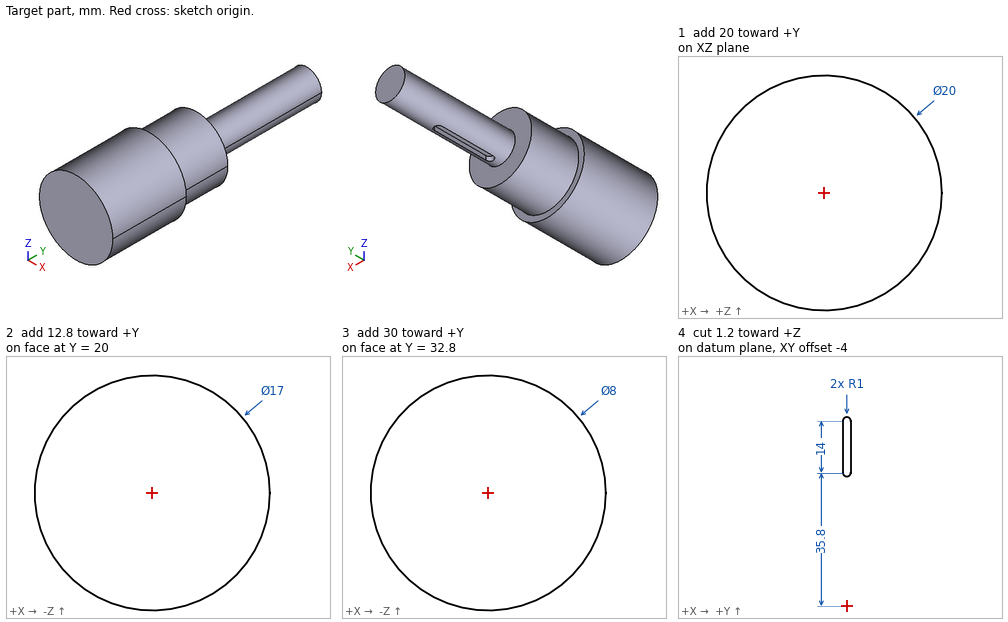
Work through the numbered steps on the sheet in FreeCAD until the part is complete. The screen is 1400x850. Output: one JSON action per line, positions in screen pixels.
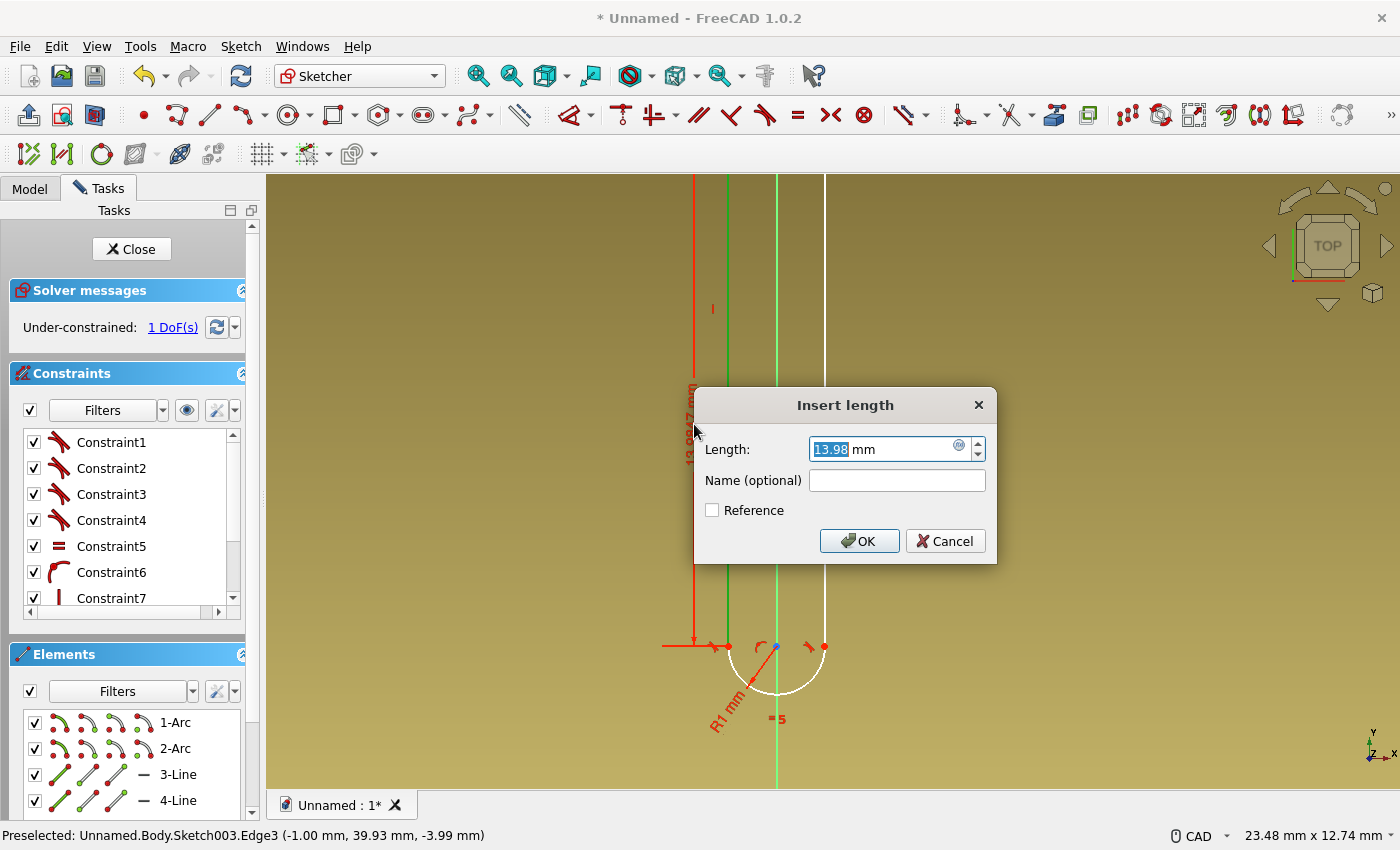
{"action": "type", "text": "14"}
{"action": "key", "text": "Return"}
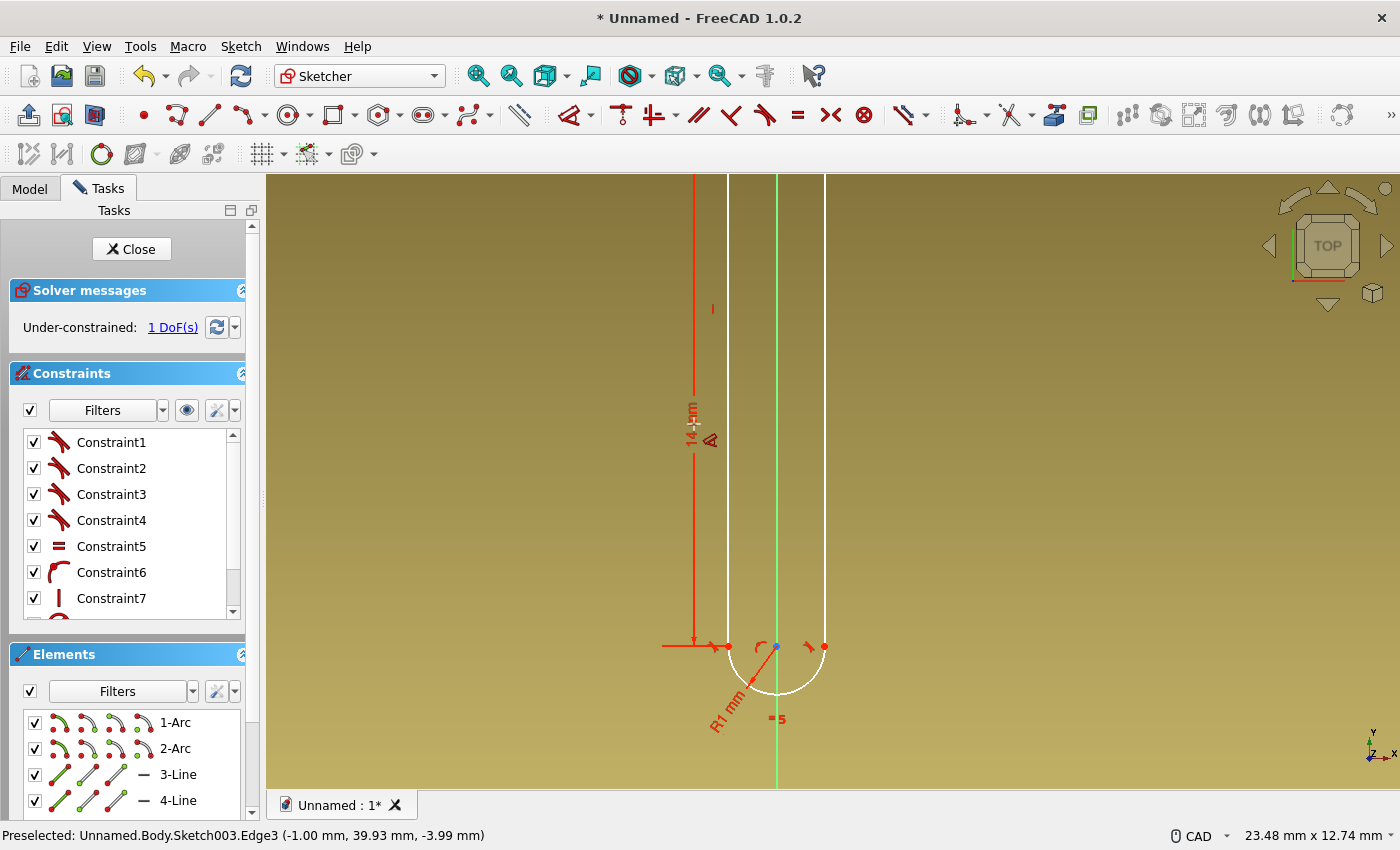
{"action": "left_click", "coordinate": [728, 646]}
{"action": "left_click", "coordinate": [694, 677]}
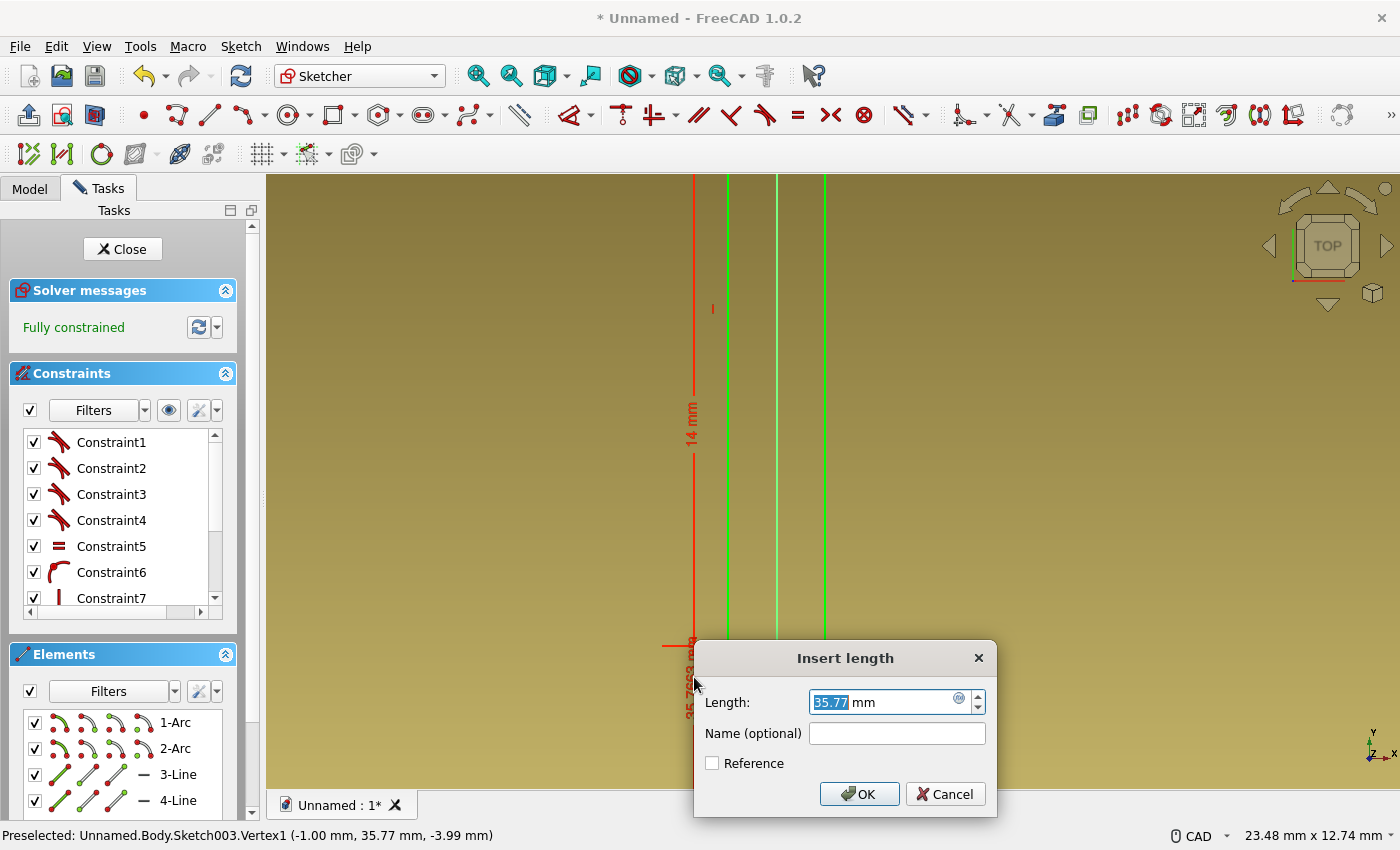
{"action": "type", "text": "35.8"}
{"action": "key", "text": "Return"}
{"action": "key", "text": "Escape"}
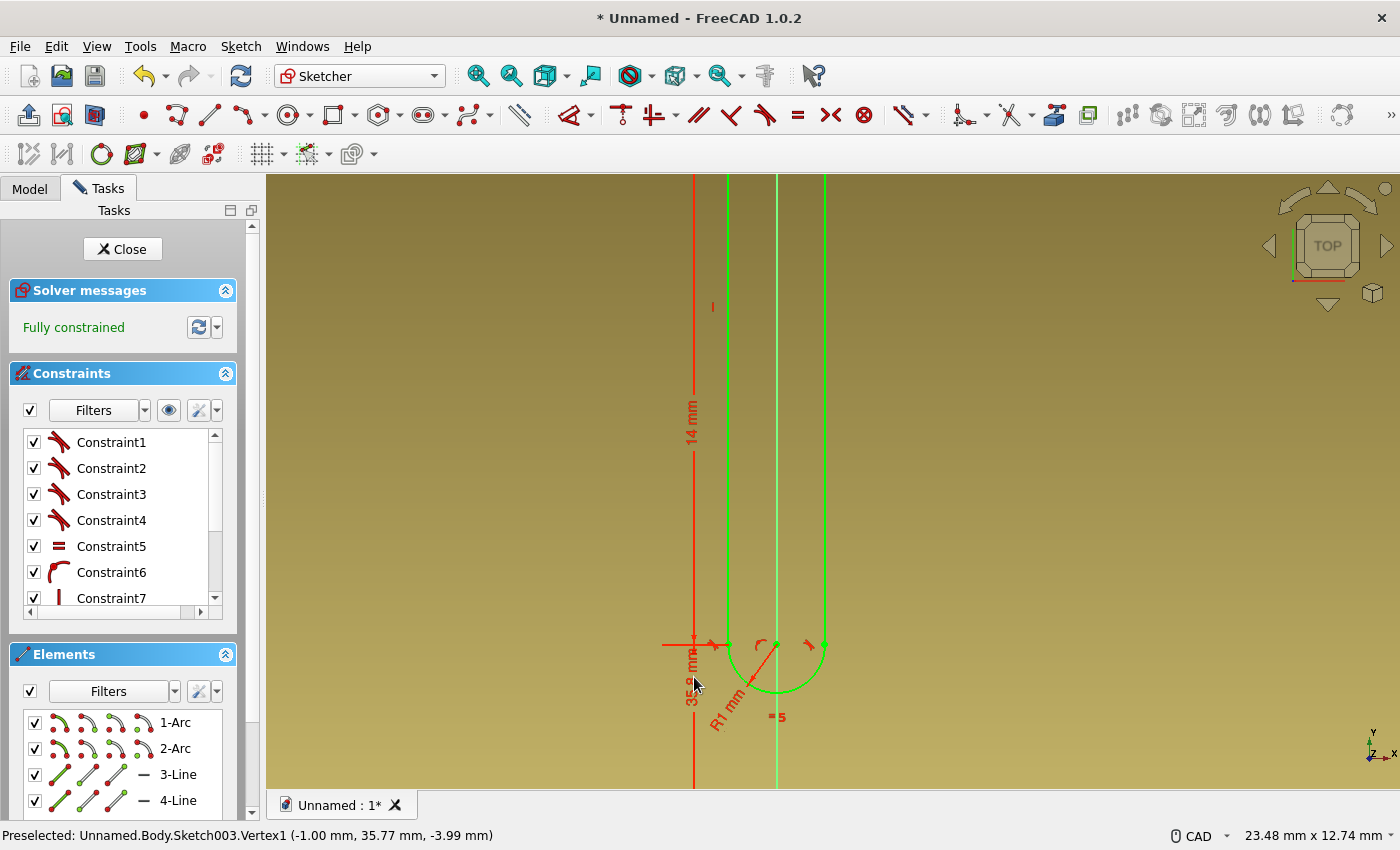
{"action": "left_click", "coordinate": [123, 249]}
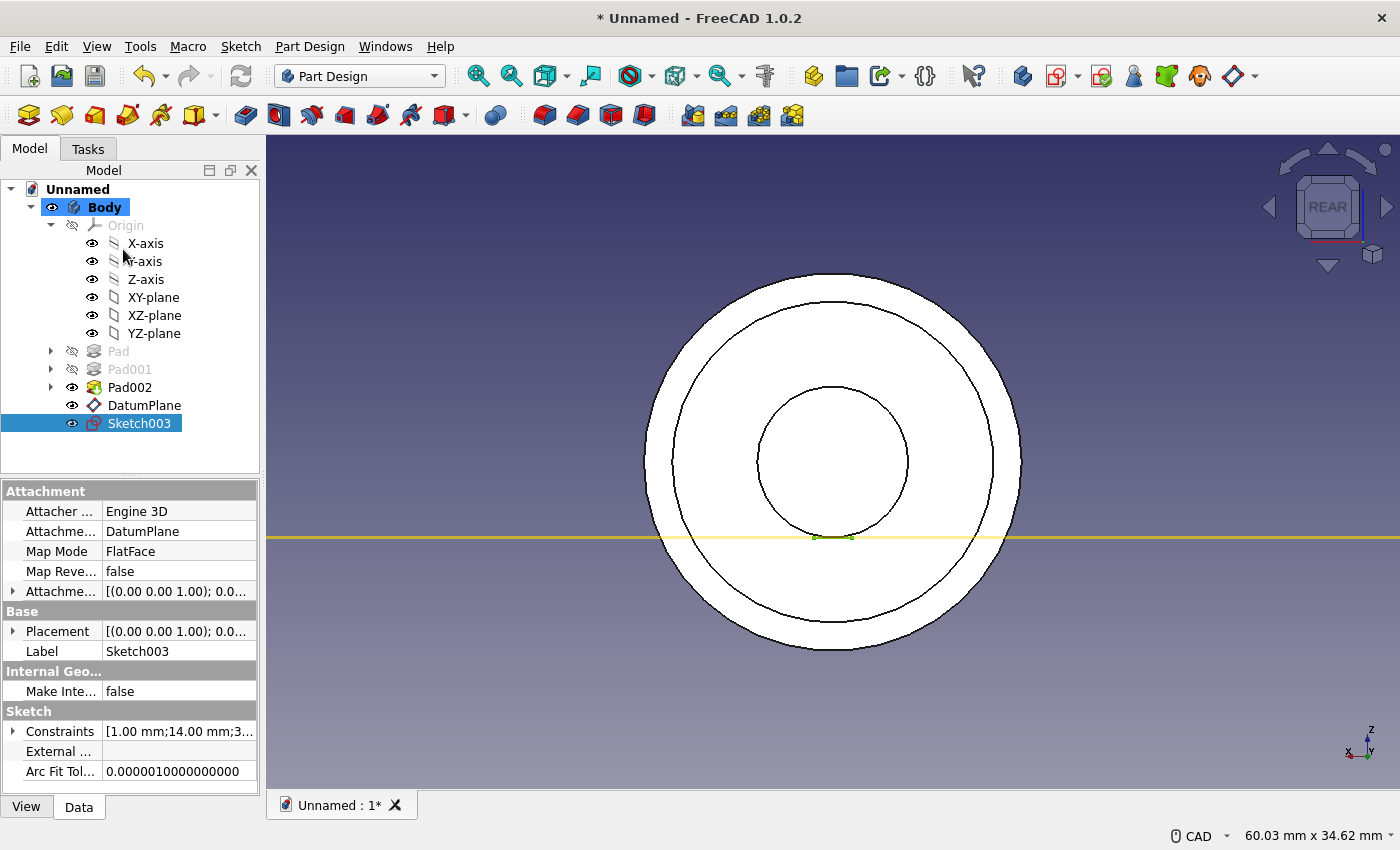
{"action": "left_click", "coordinate": [246, 116]}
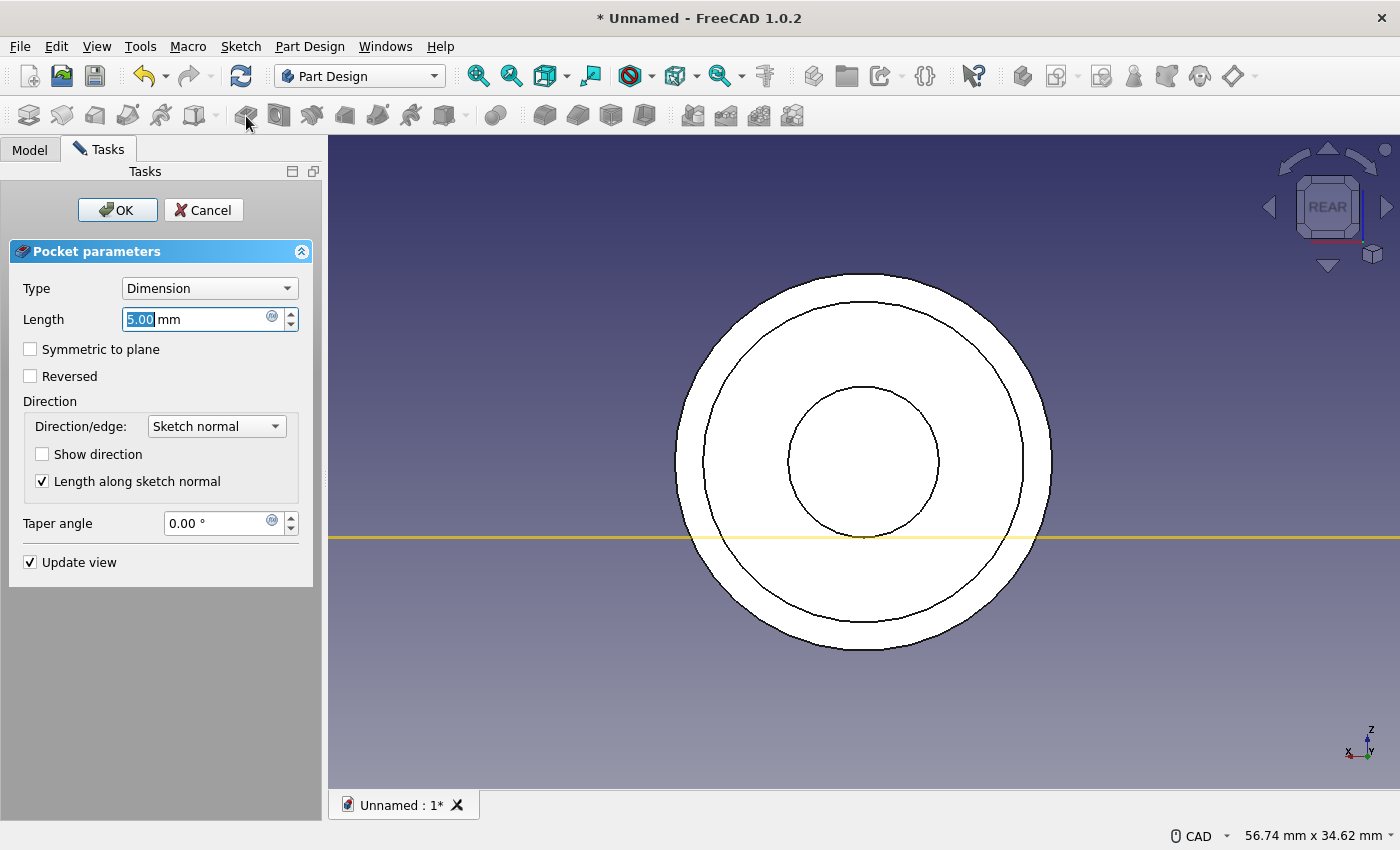
{"action": "type", "text": "1.2"}
{"action": "key", "text": "Tab"}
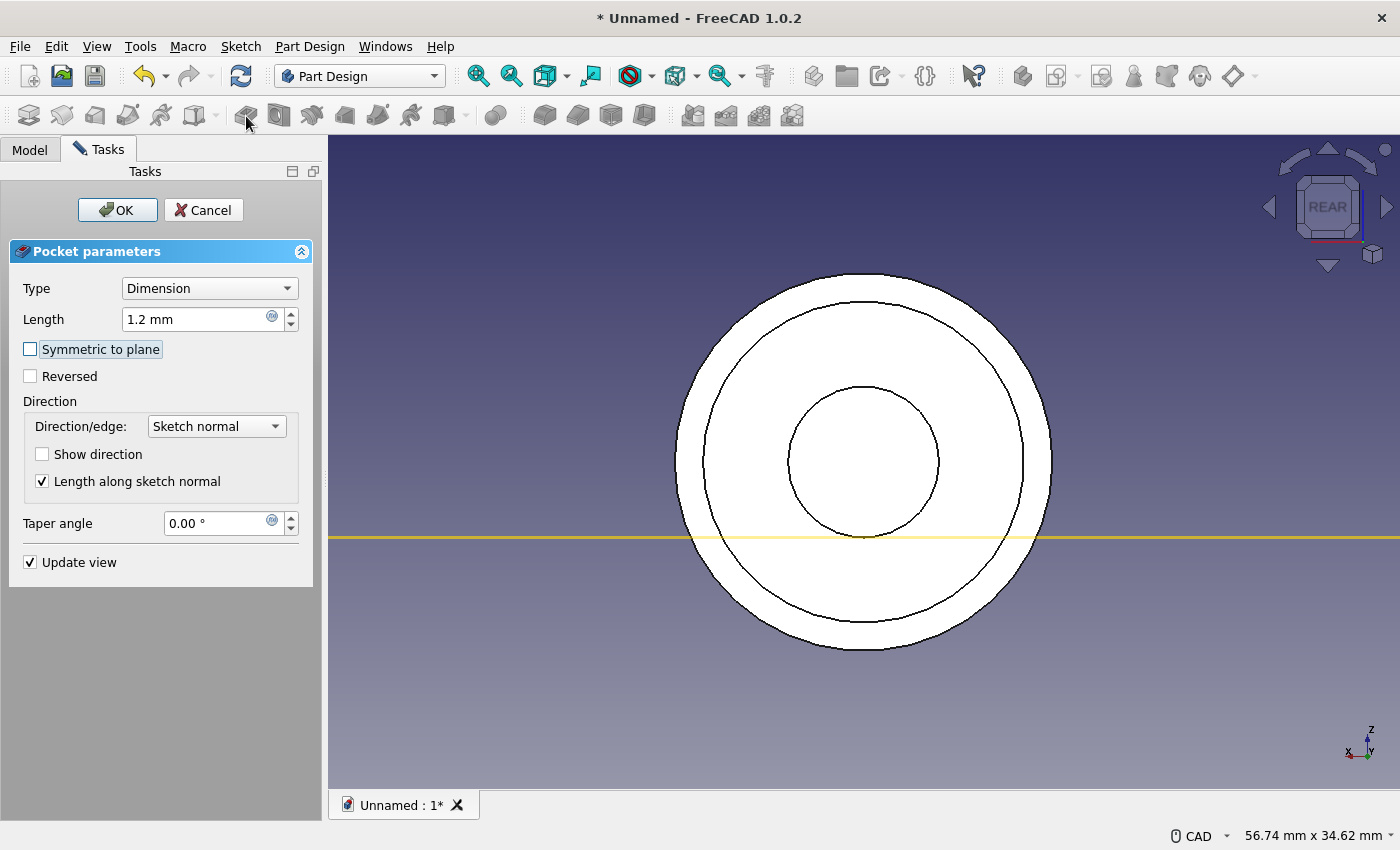
{"action": "left_click", "coordinate": [31, 376]}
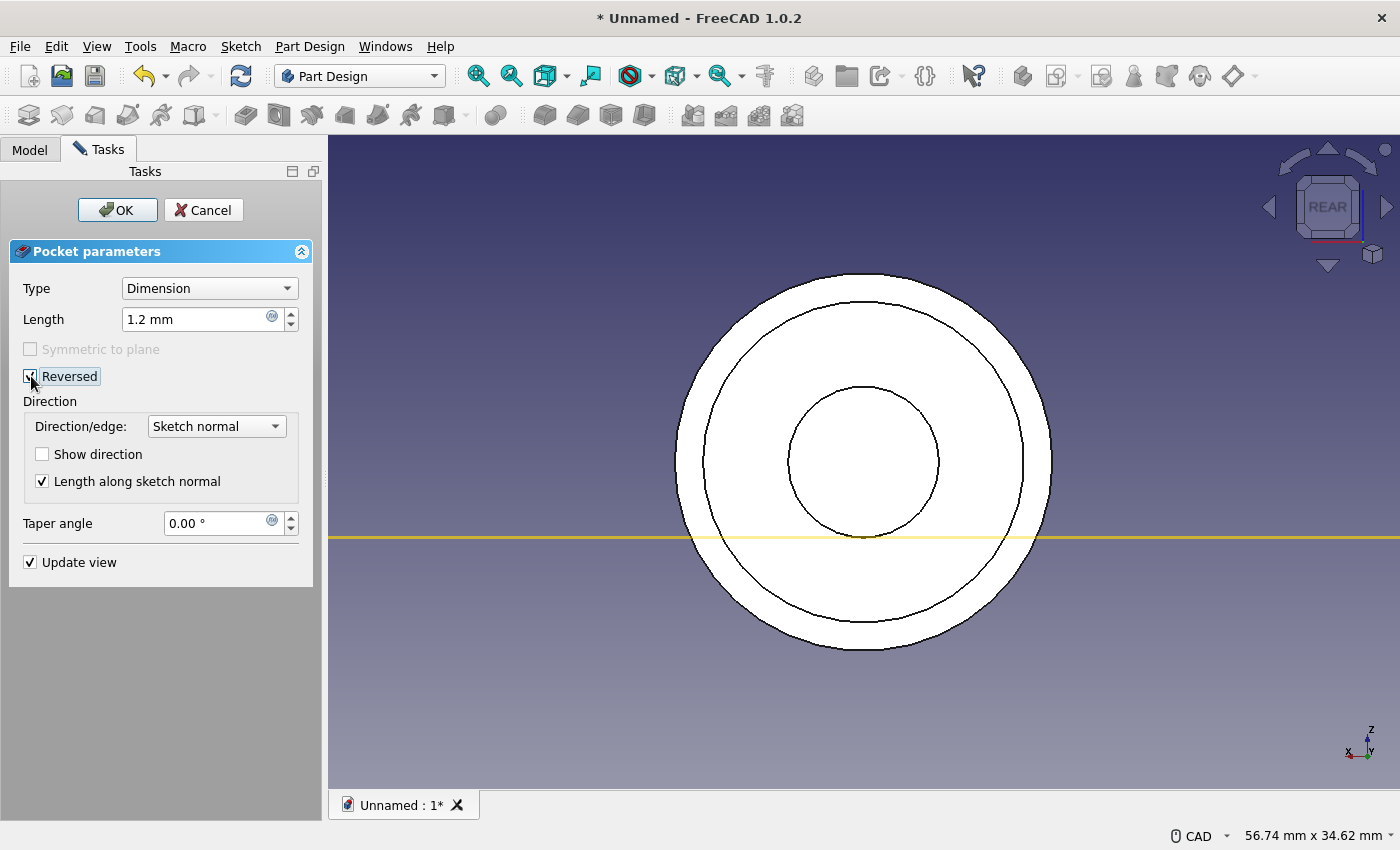
{"action": "left_click", "coordinate": [118, 210]}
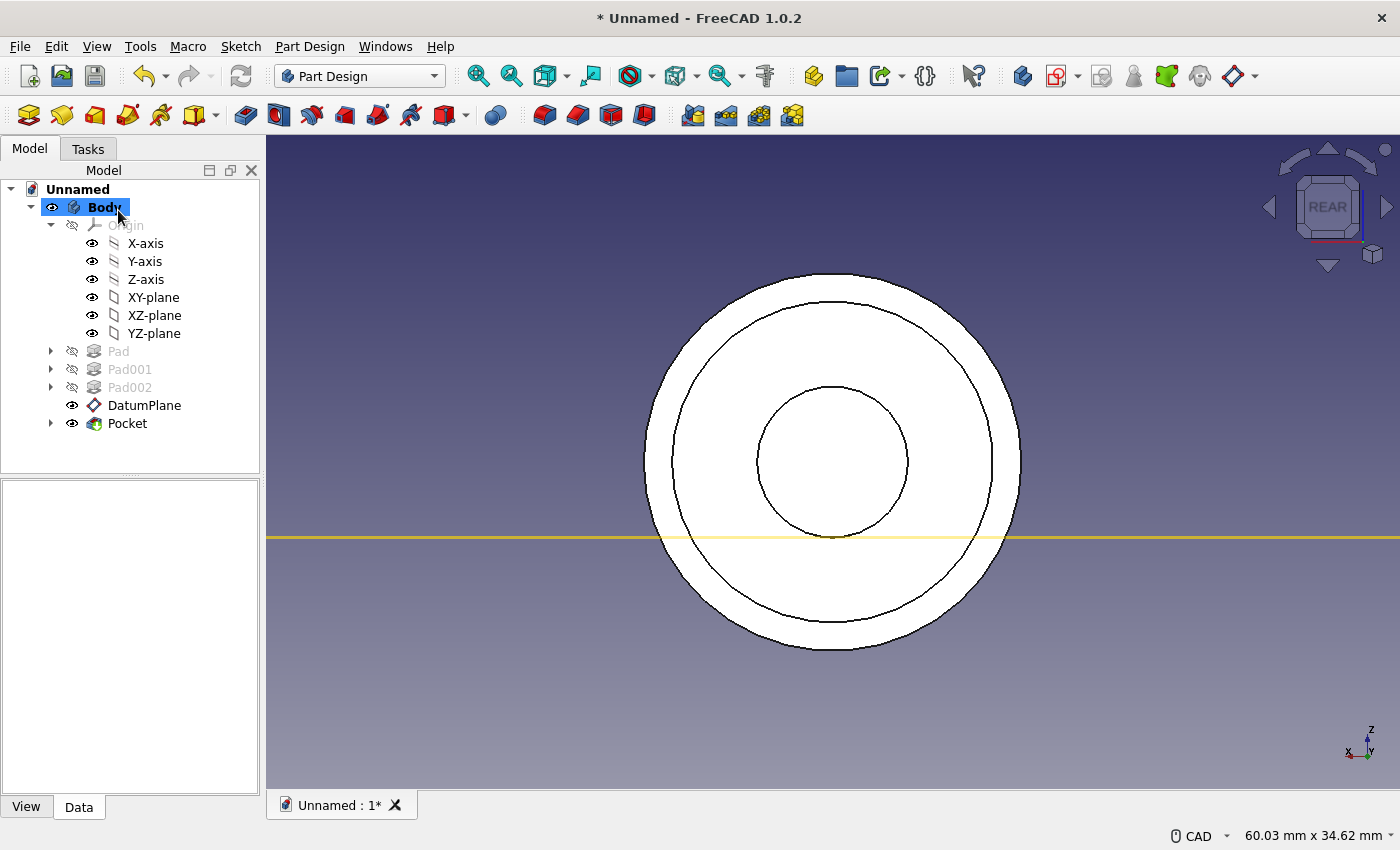
{"action": "left_click", "coordinate": [117, 405]}
{"action": "key", "text": "space"}